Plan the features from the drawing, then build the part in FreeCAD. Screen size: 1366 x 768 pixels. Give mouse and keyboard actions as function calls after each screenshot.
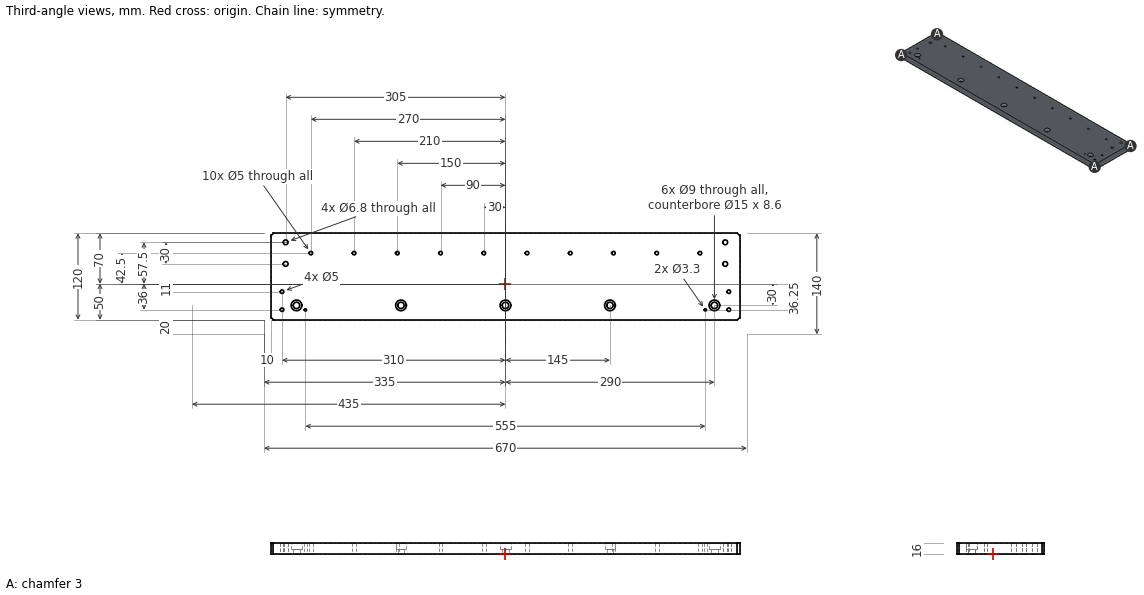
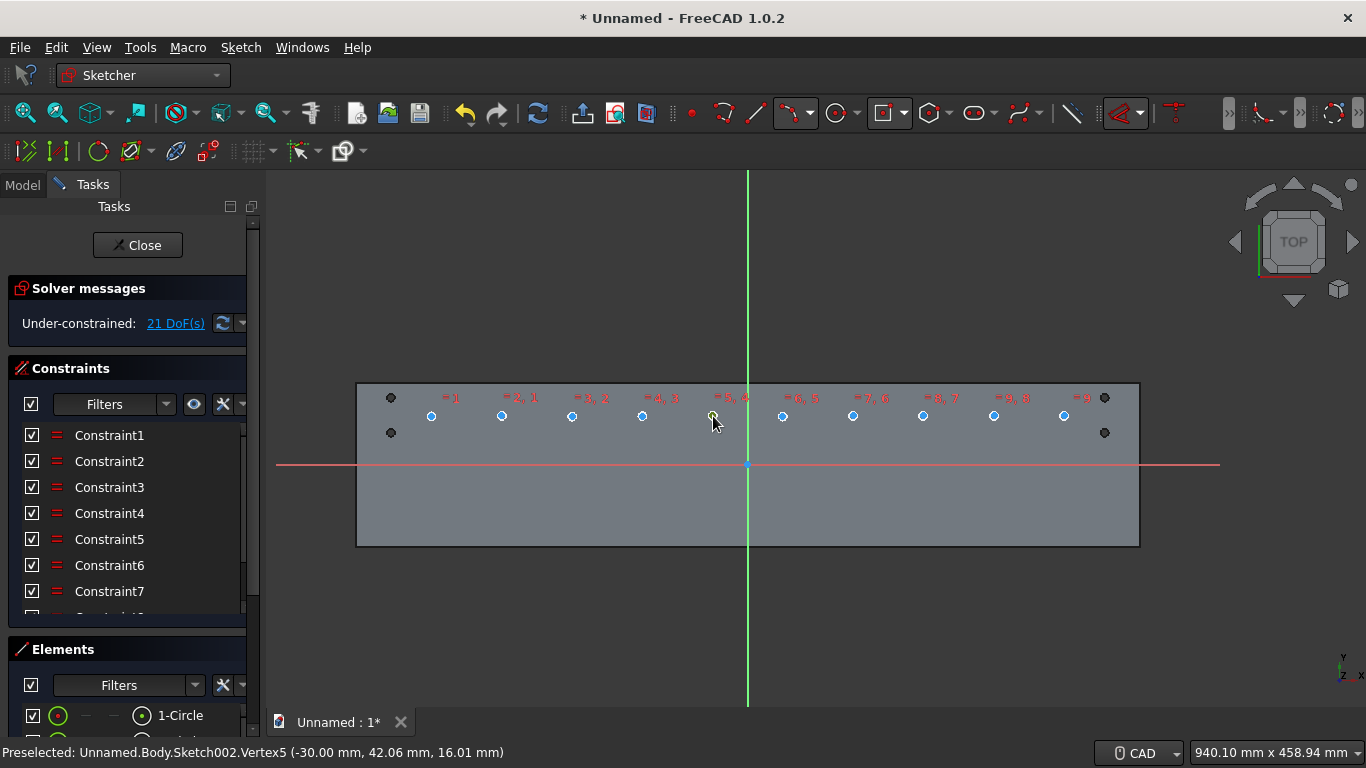
click(783, 417)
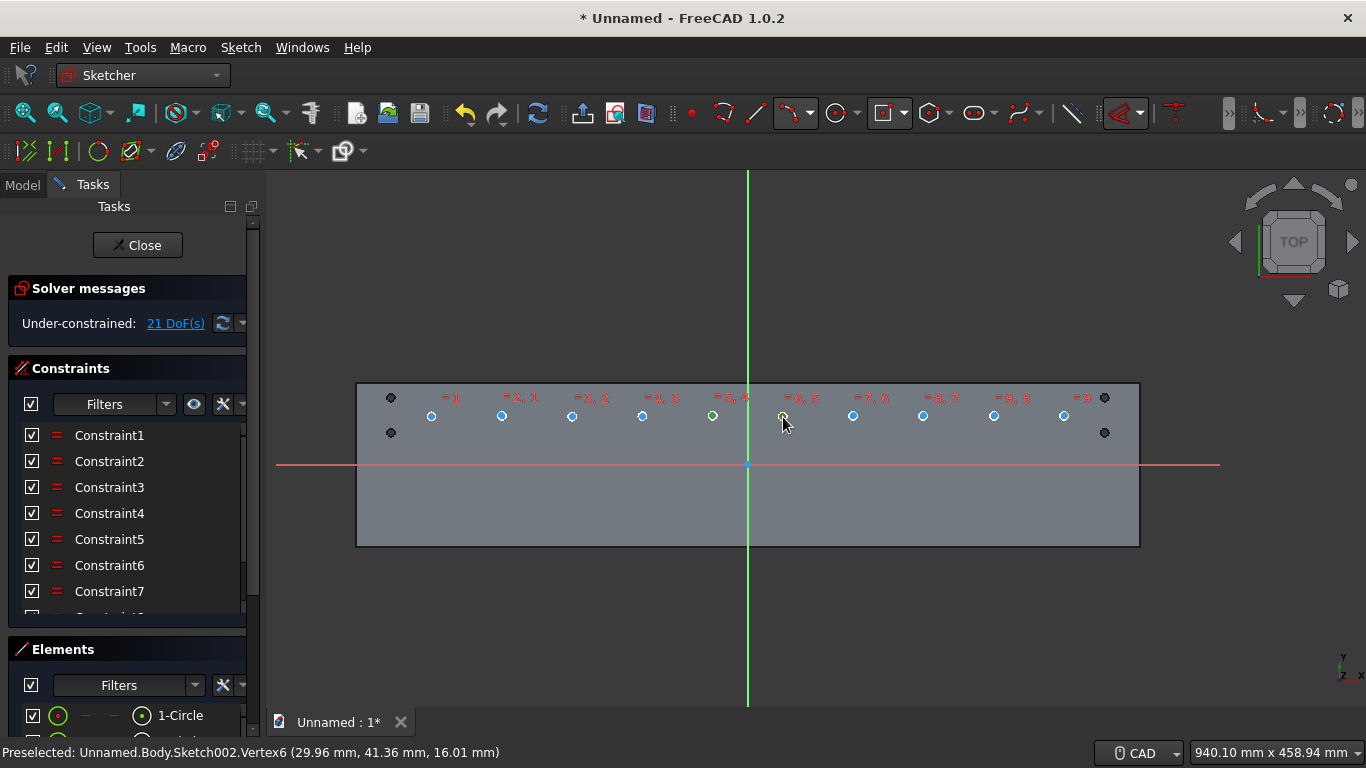
click(748, 645)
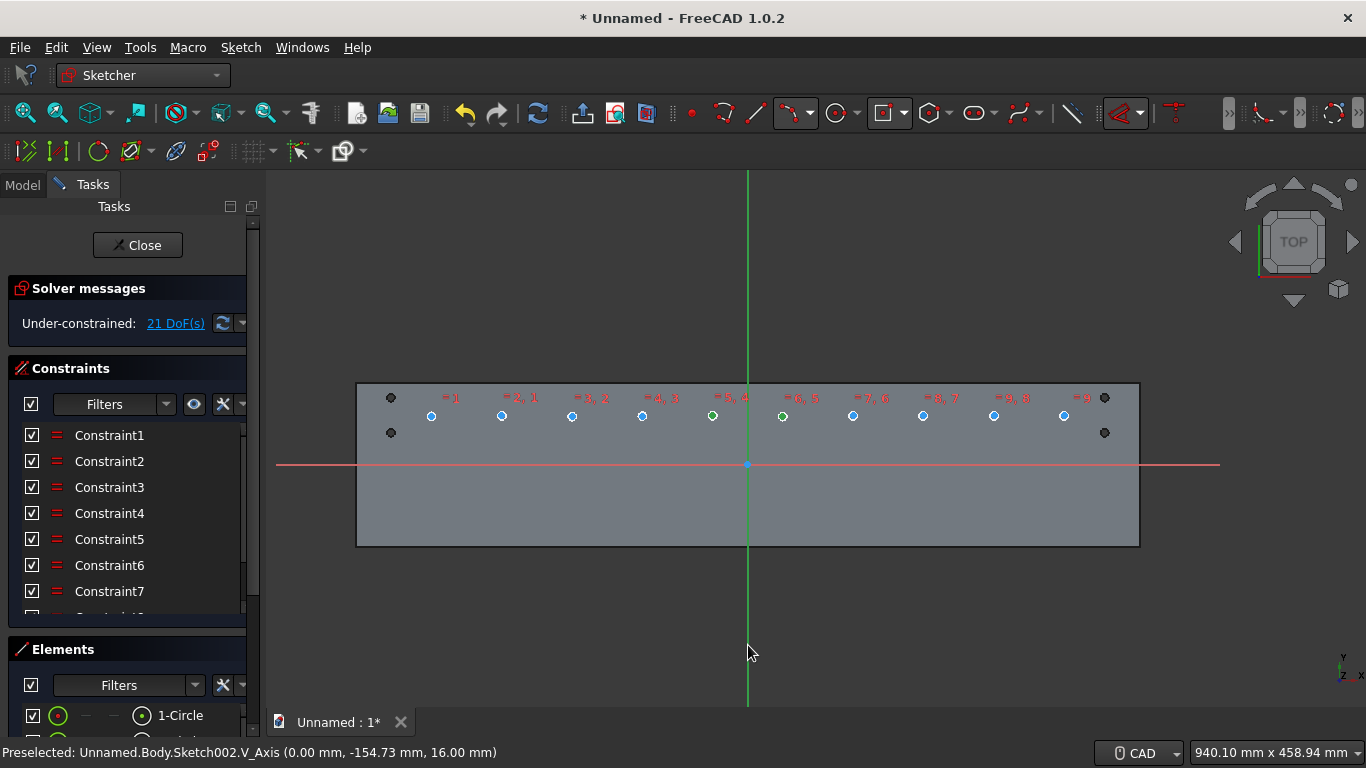
key(s)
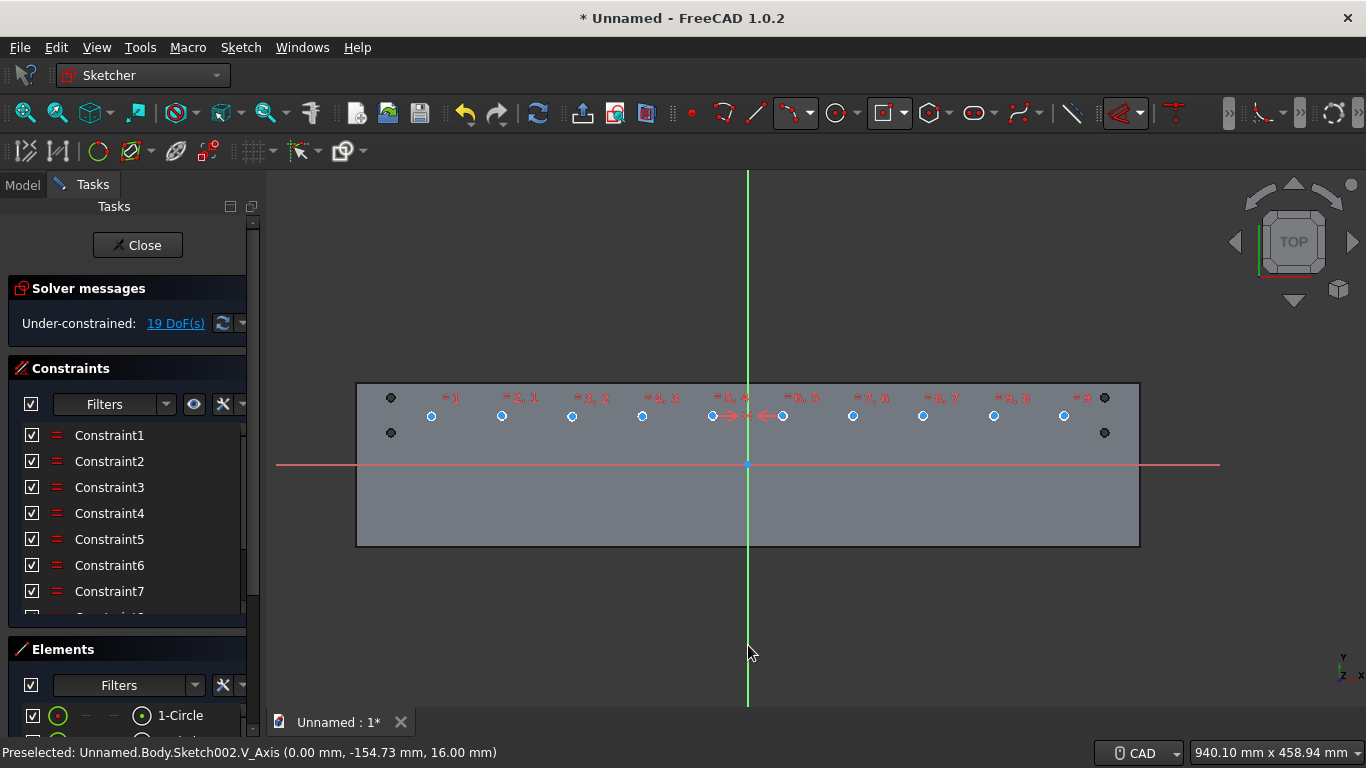
click(642, 416)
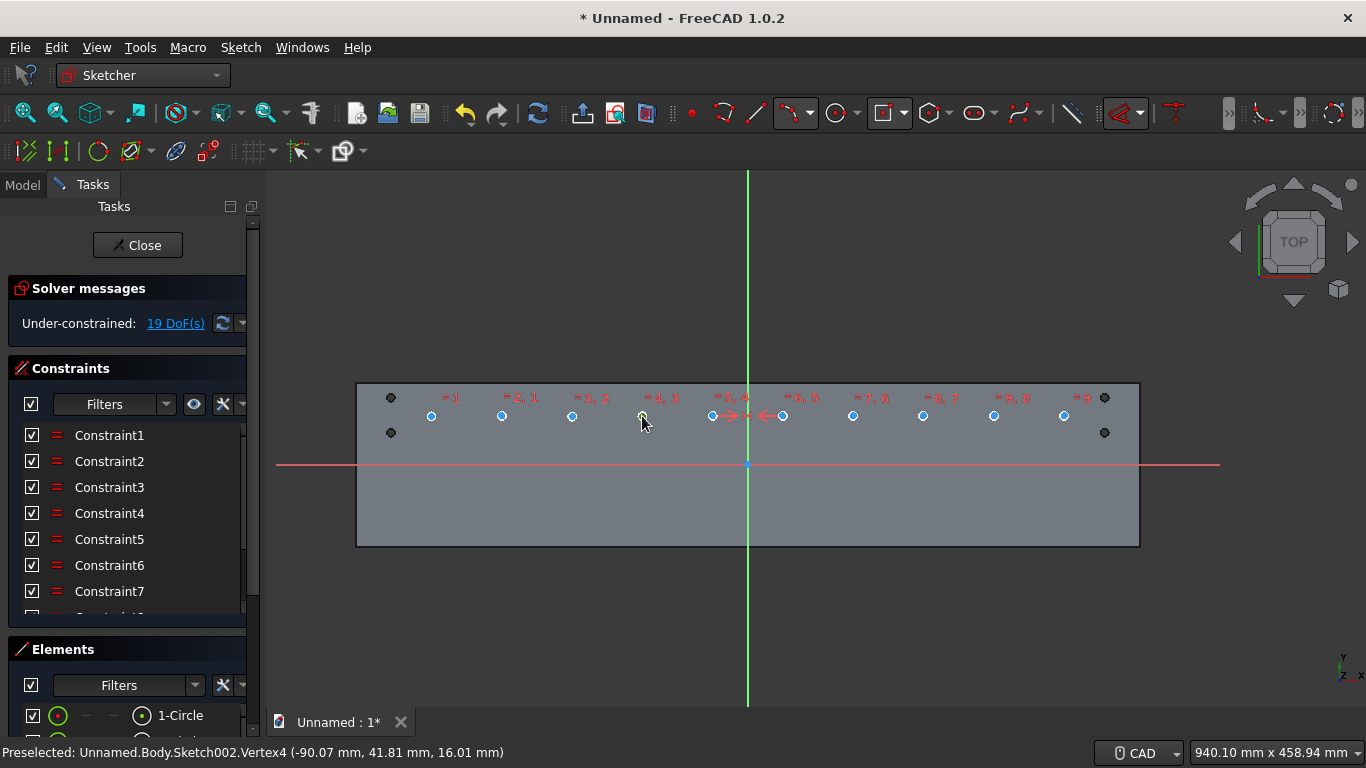
click(853, 416)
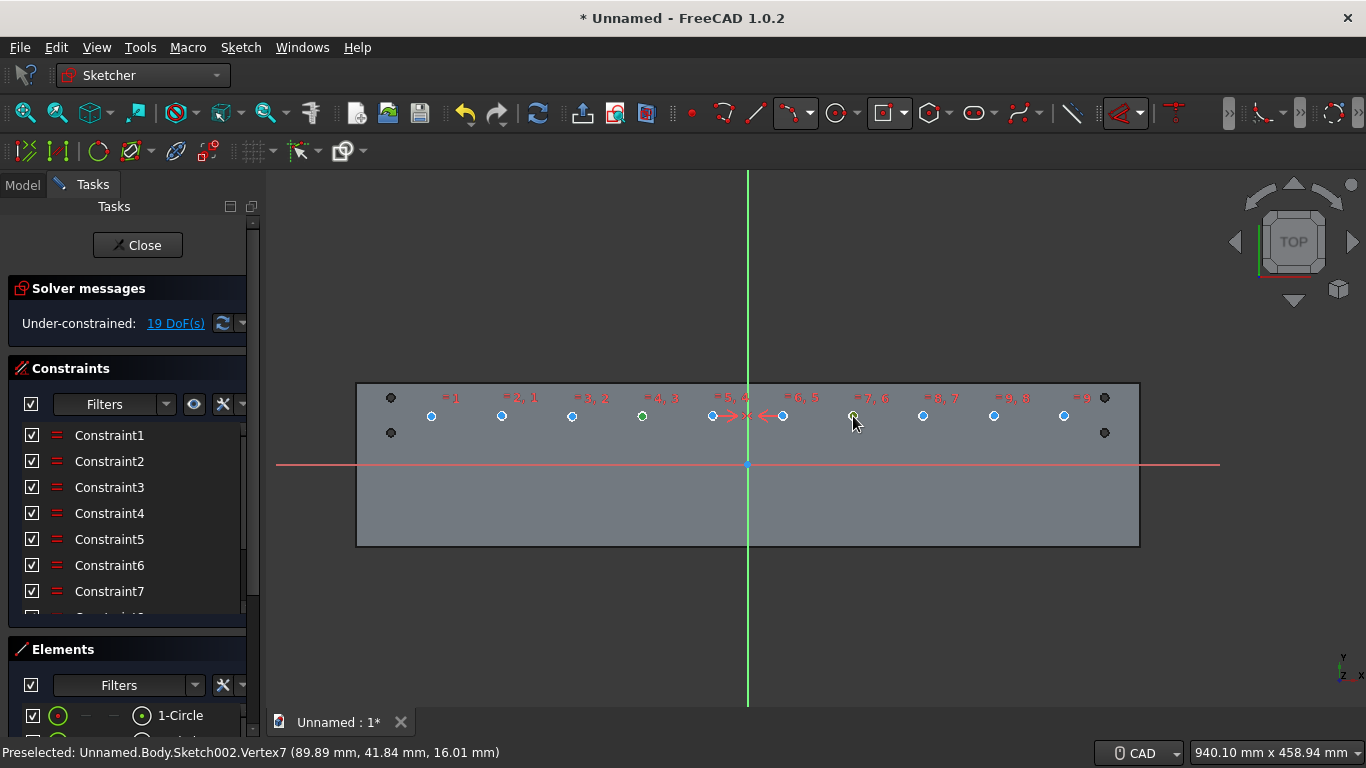
click(748, 645)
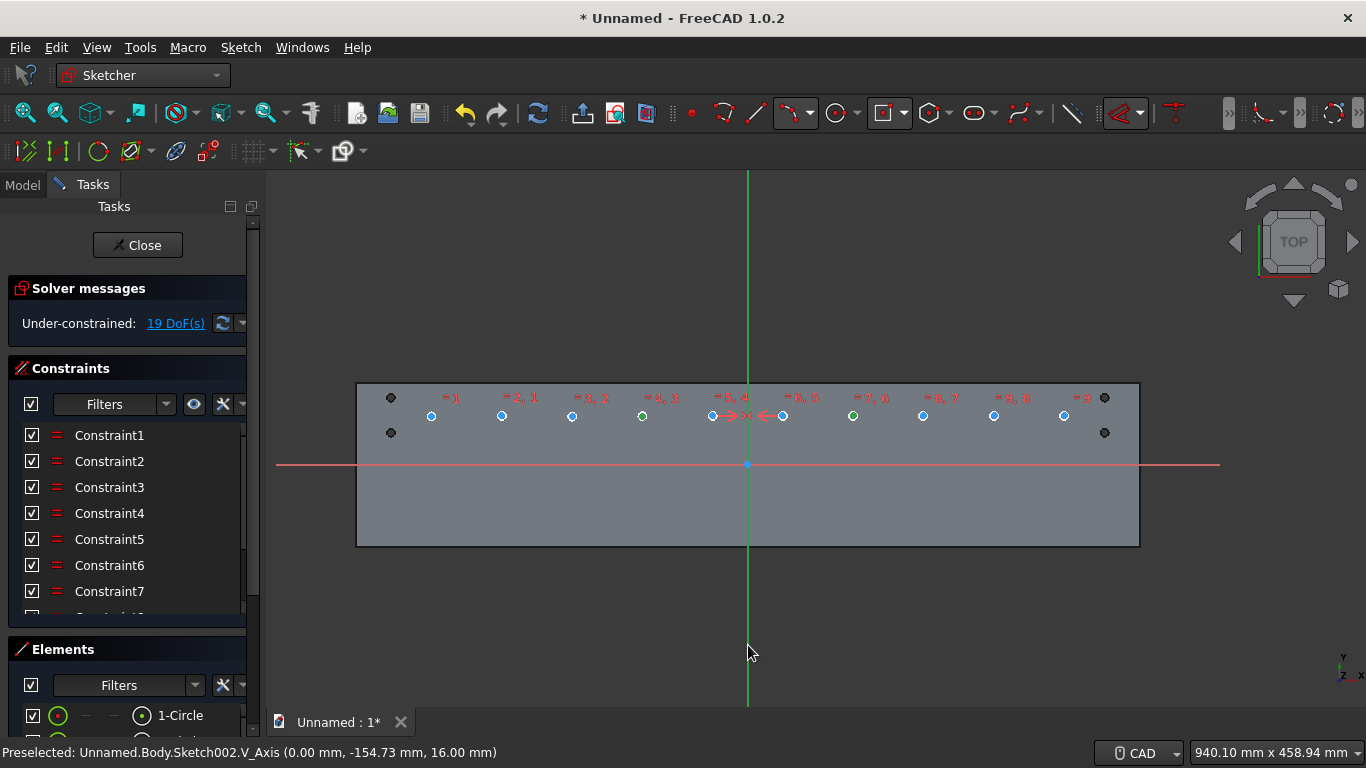
key(s)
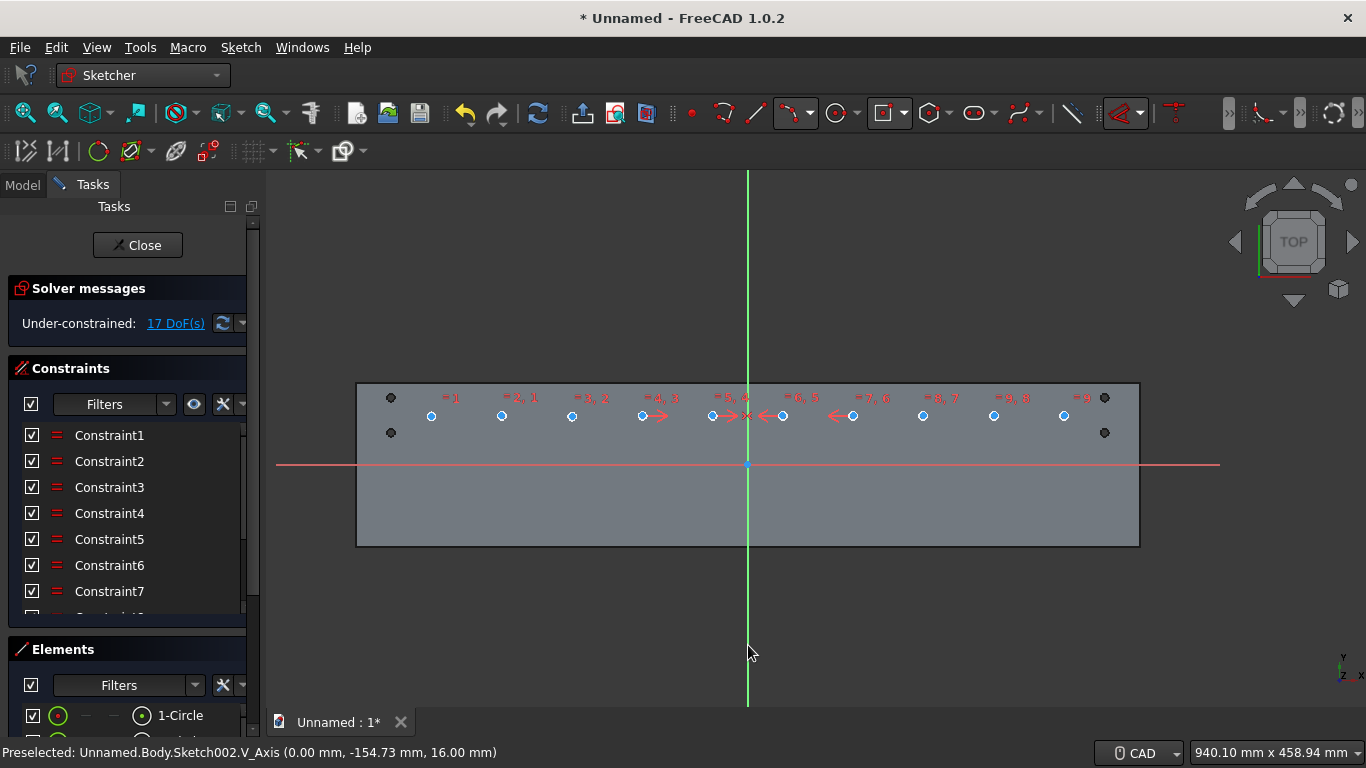
click(572, 417)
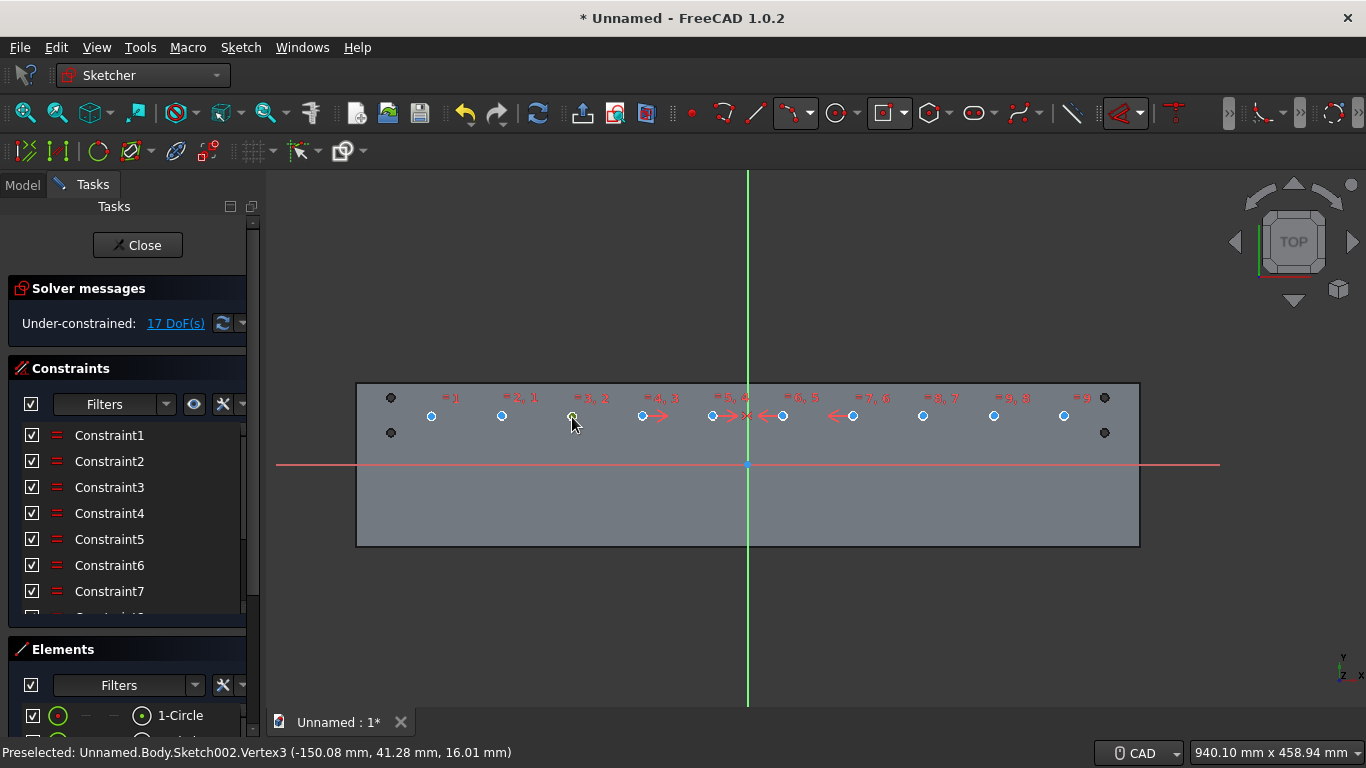
click(923, 416)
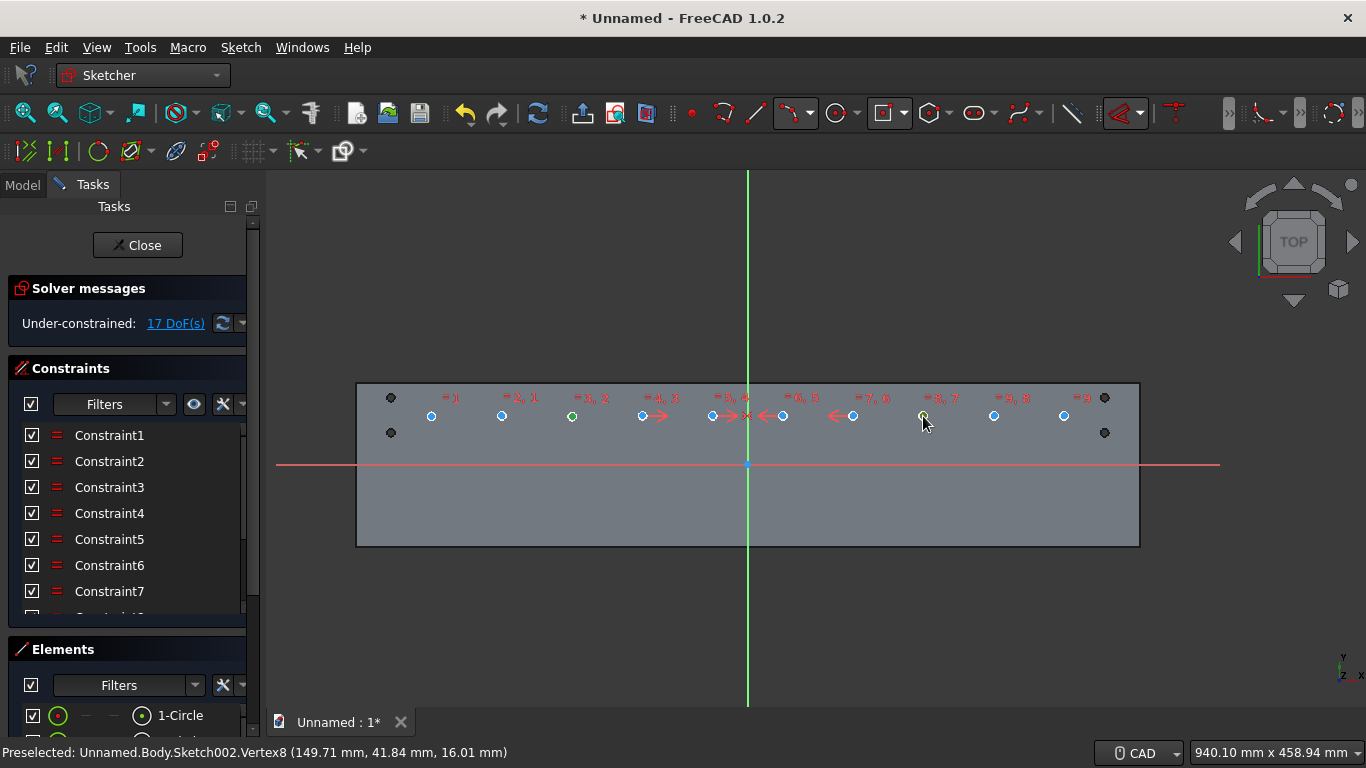
click(748, 645)